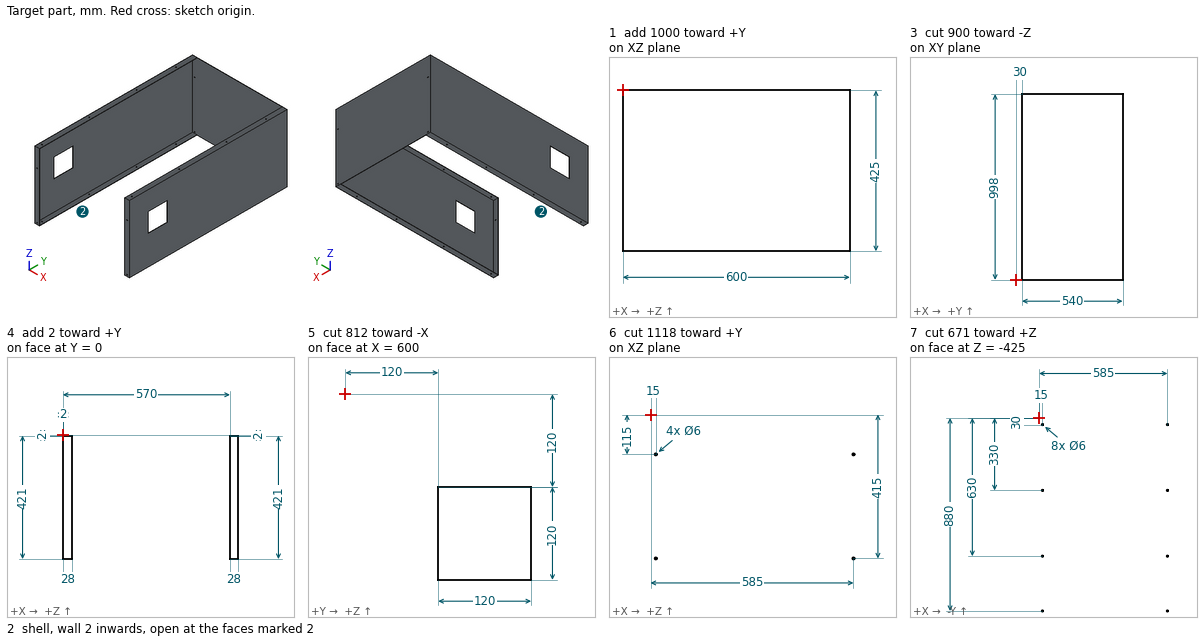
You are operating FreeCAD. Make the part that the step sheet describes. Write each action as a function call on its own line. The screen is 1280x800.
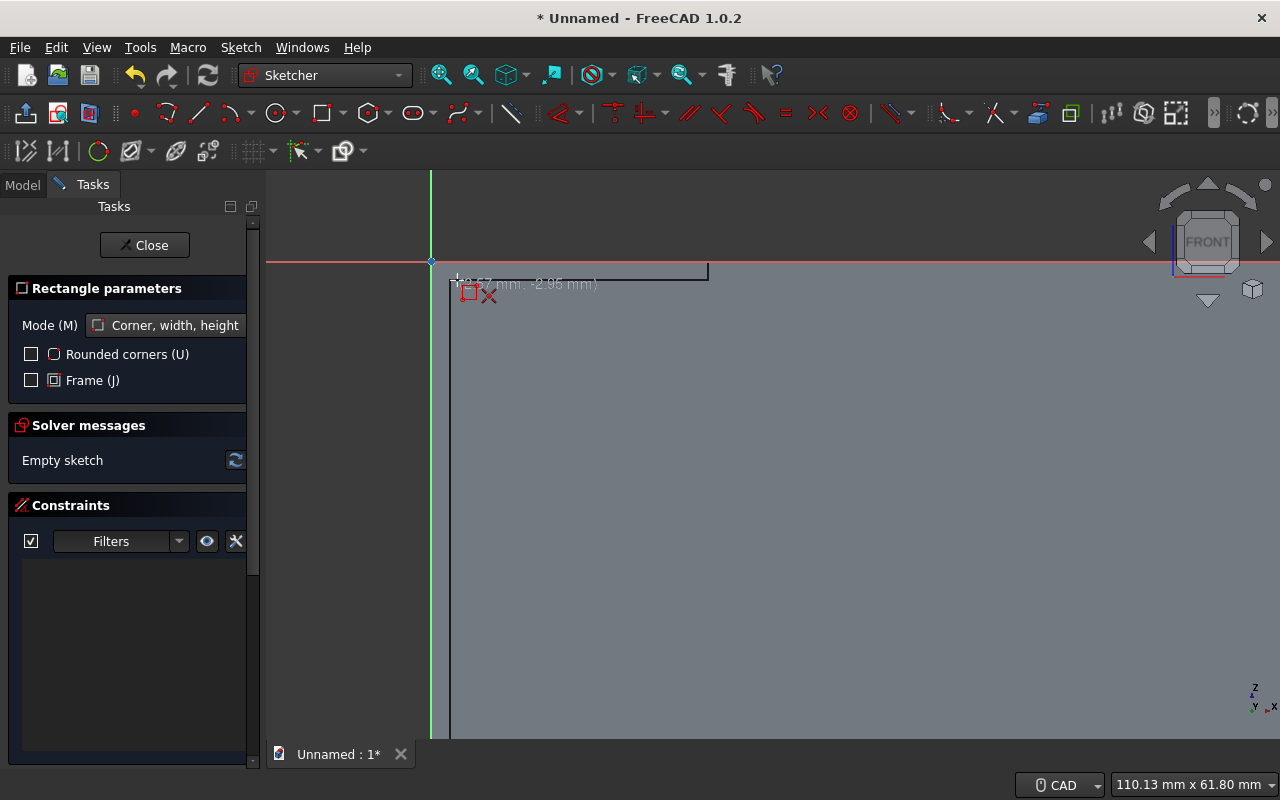
click(450, 280)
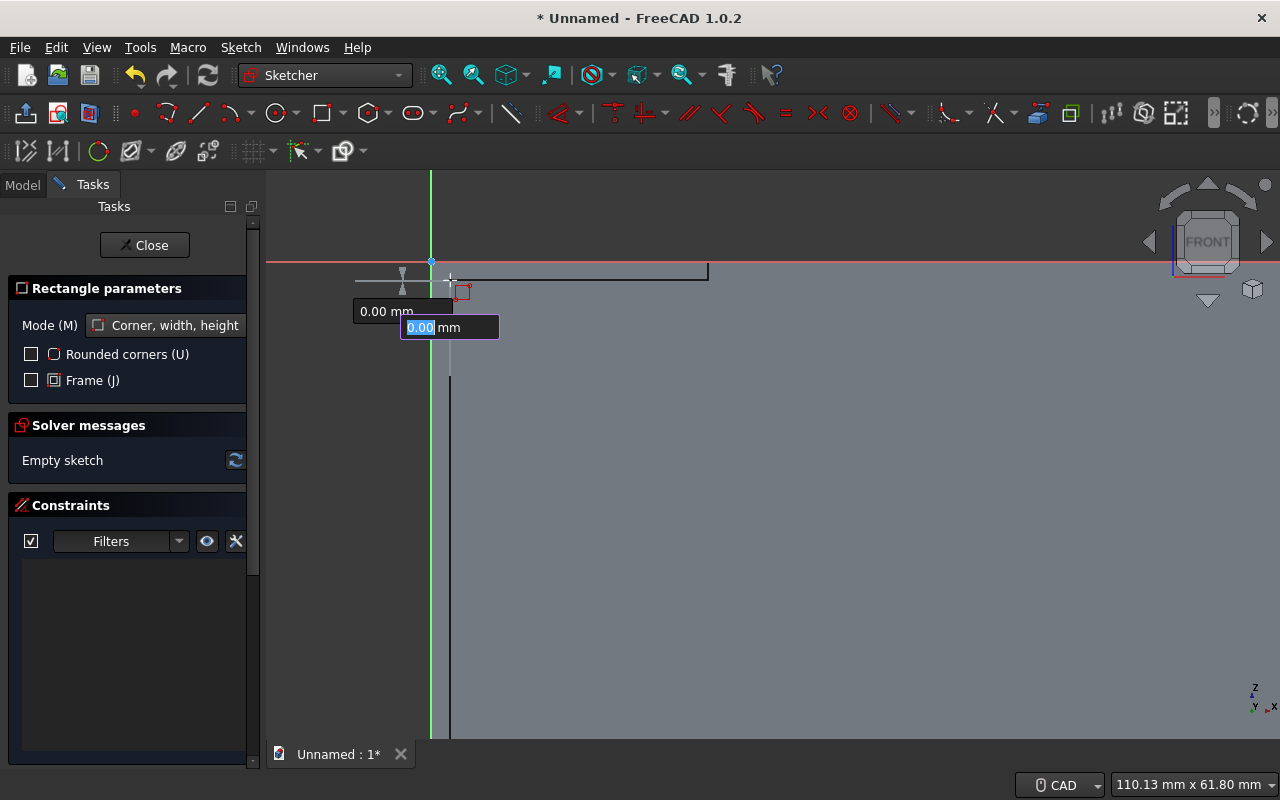
scroll(457, 279, down, 12)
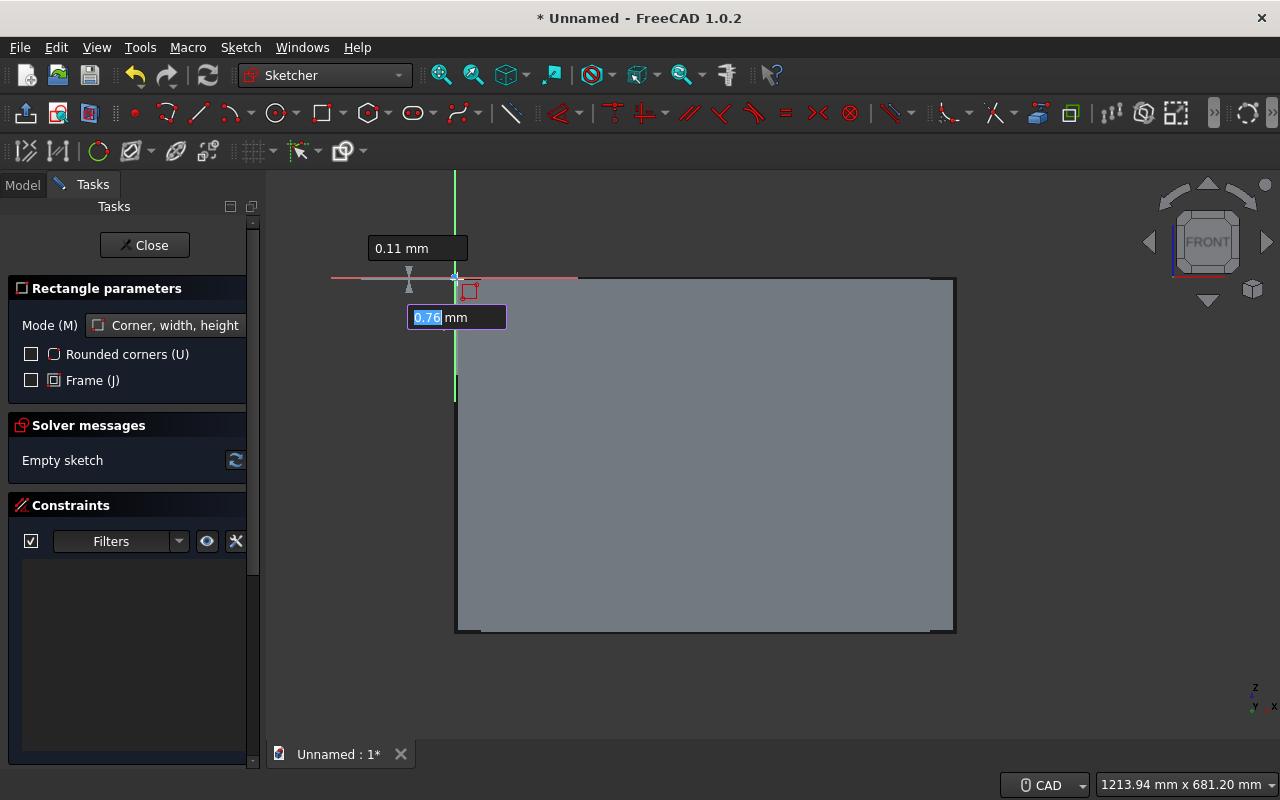
click(480, 631)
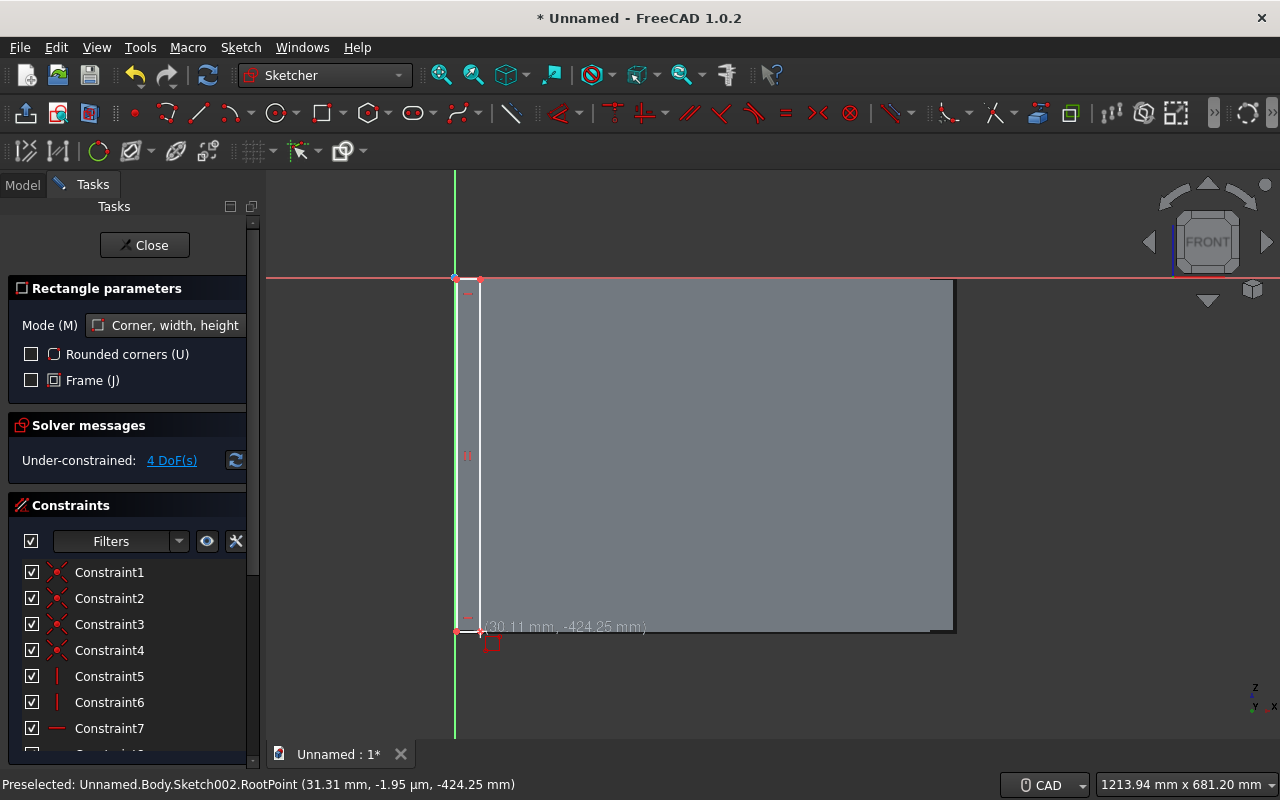
scroll(931, 279, up, 12)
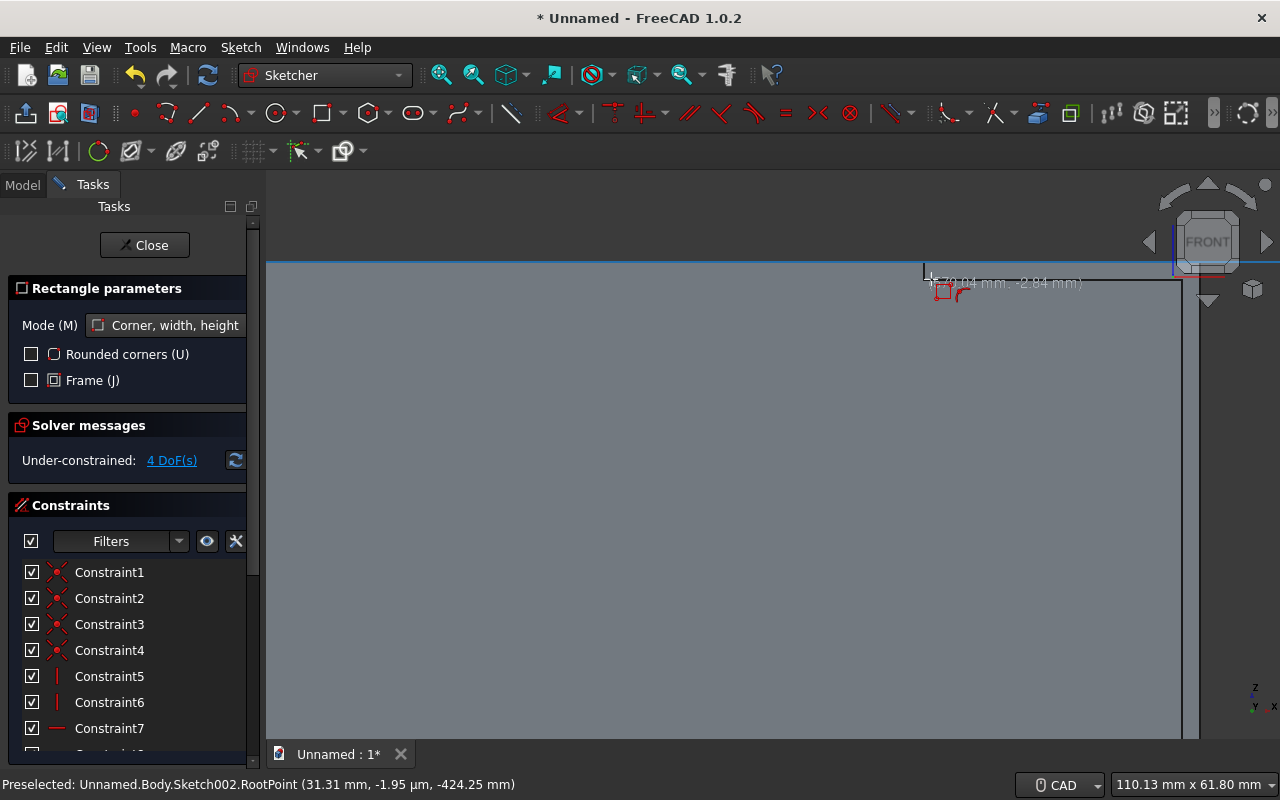
click(924, 280)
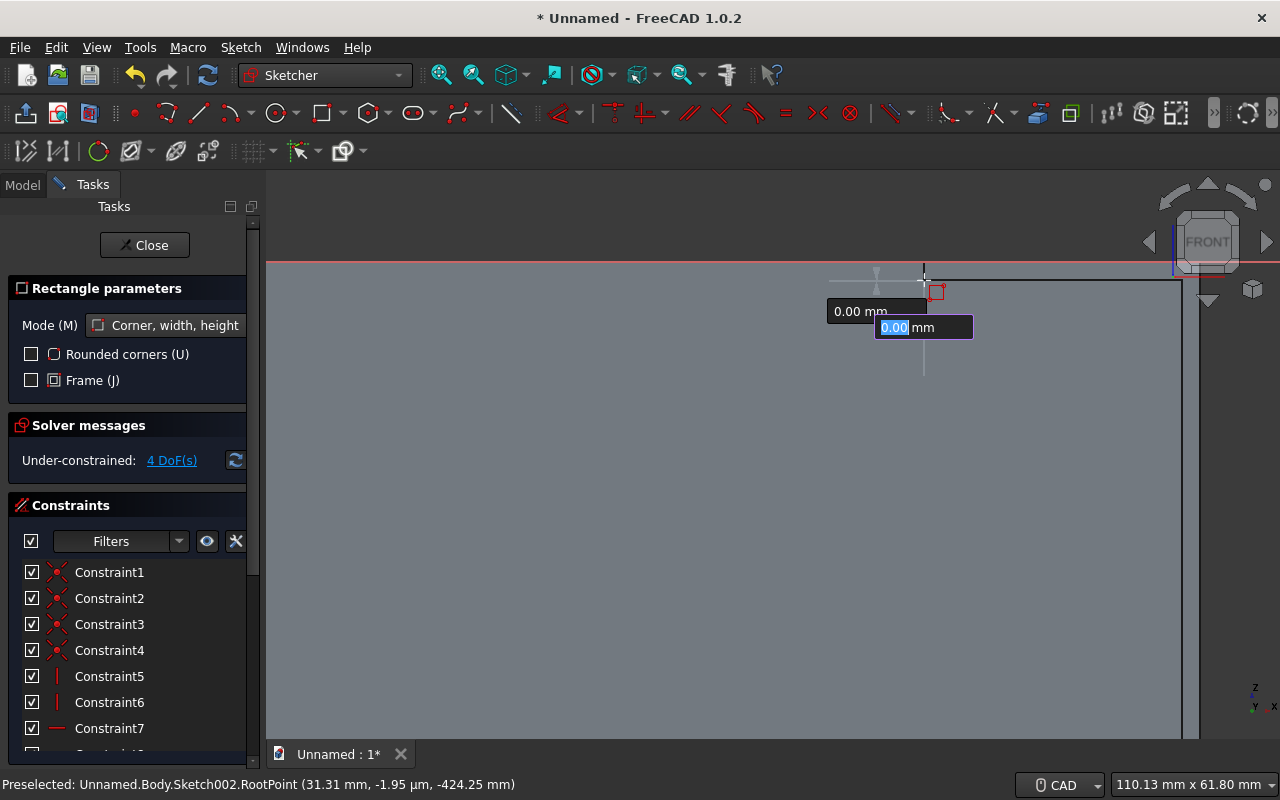
scroll(932, 279, down, 12)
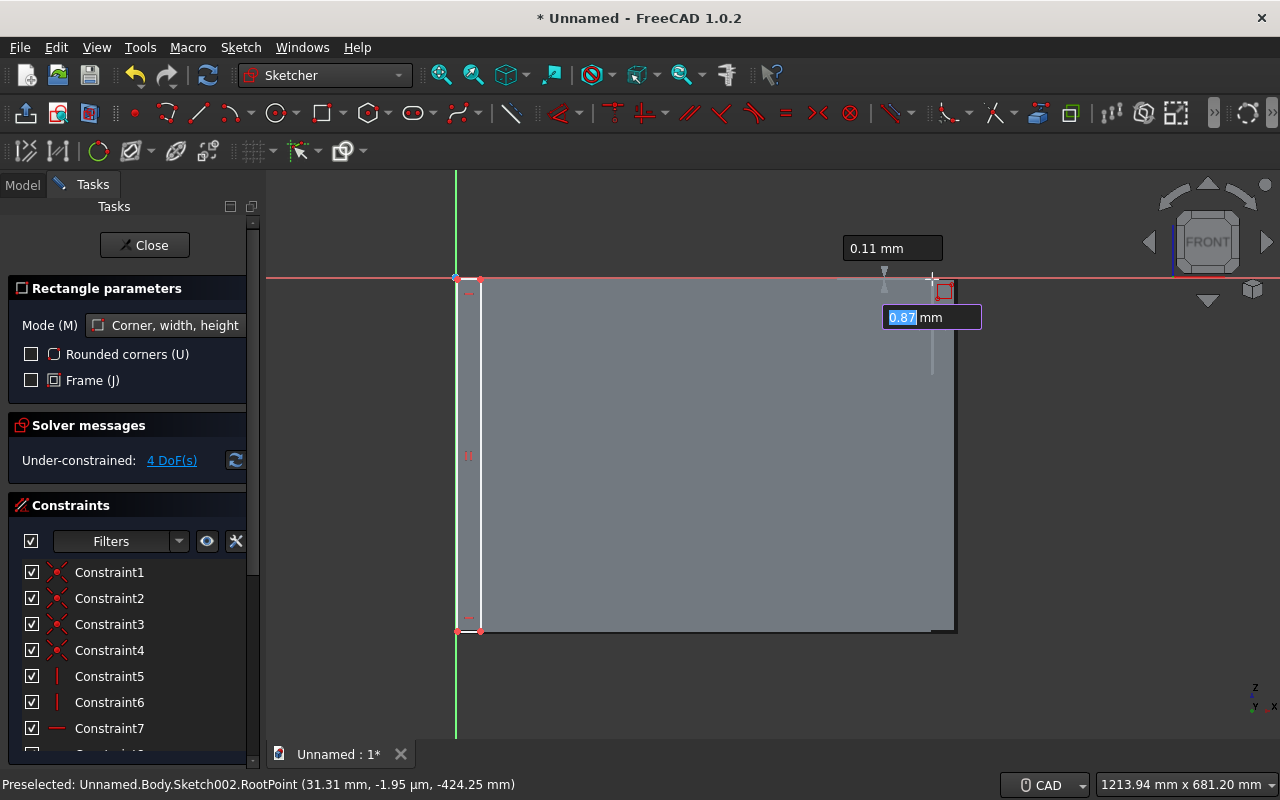
click(955, 631)
key(Escape)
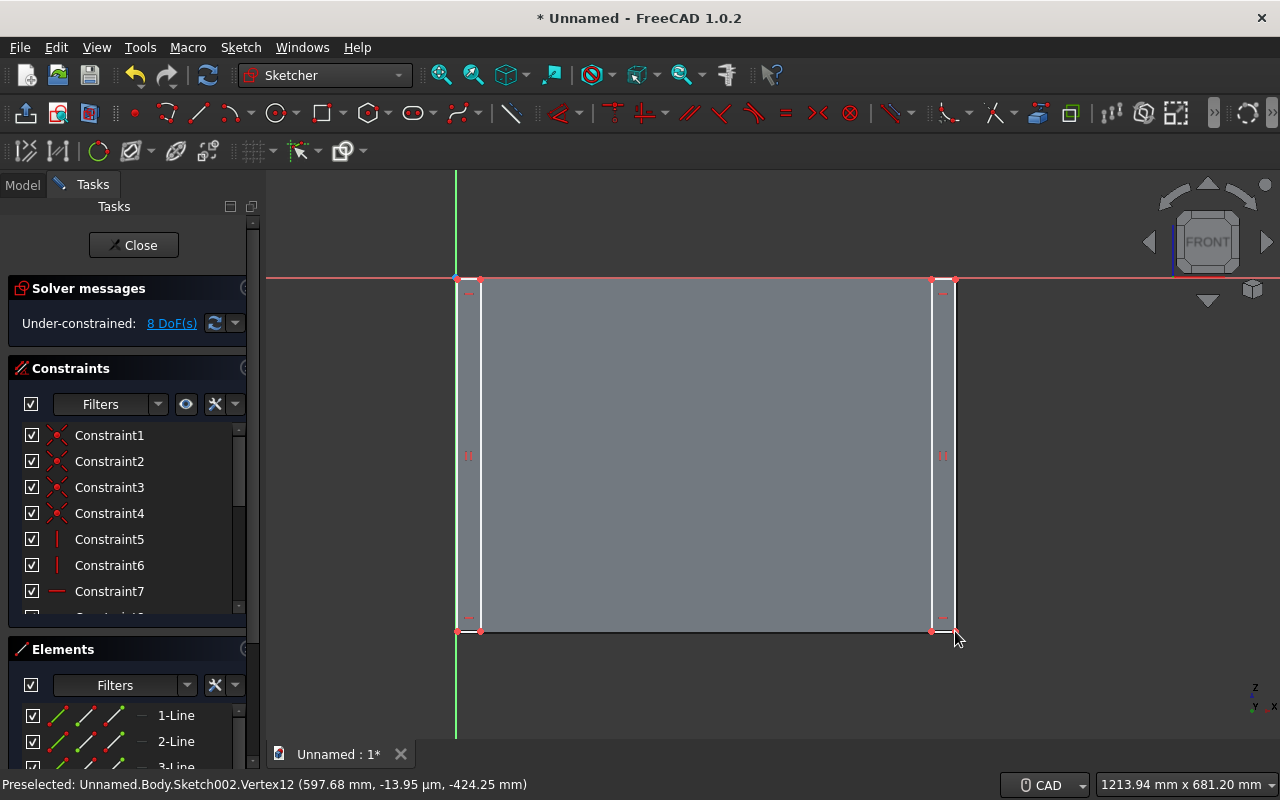
scroll(467, 632, up, 3)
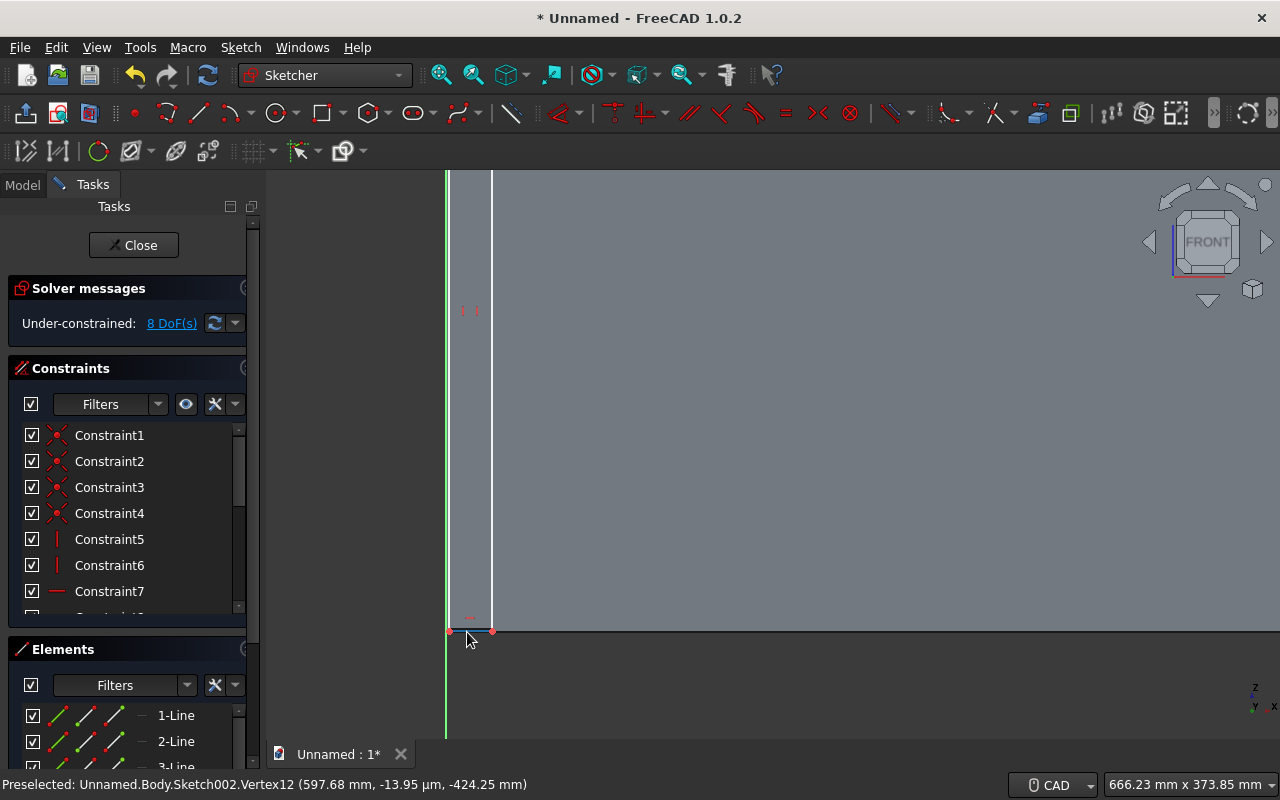
click(467, 631)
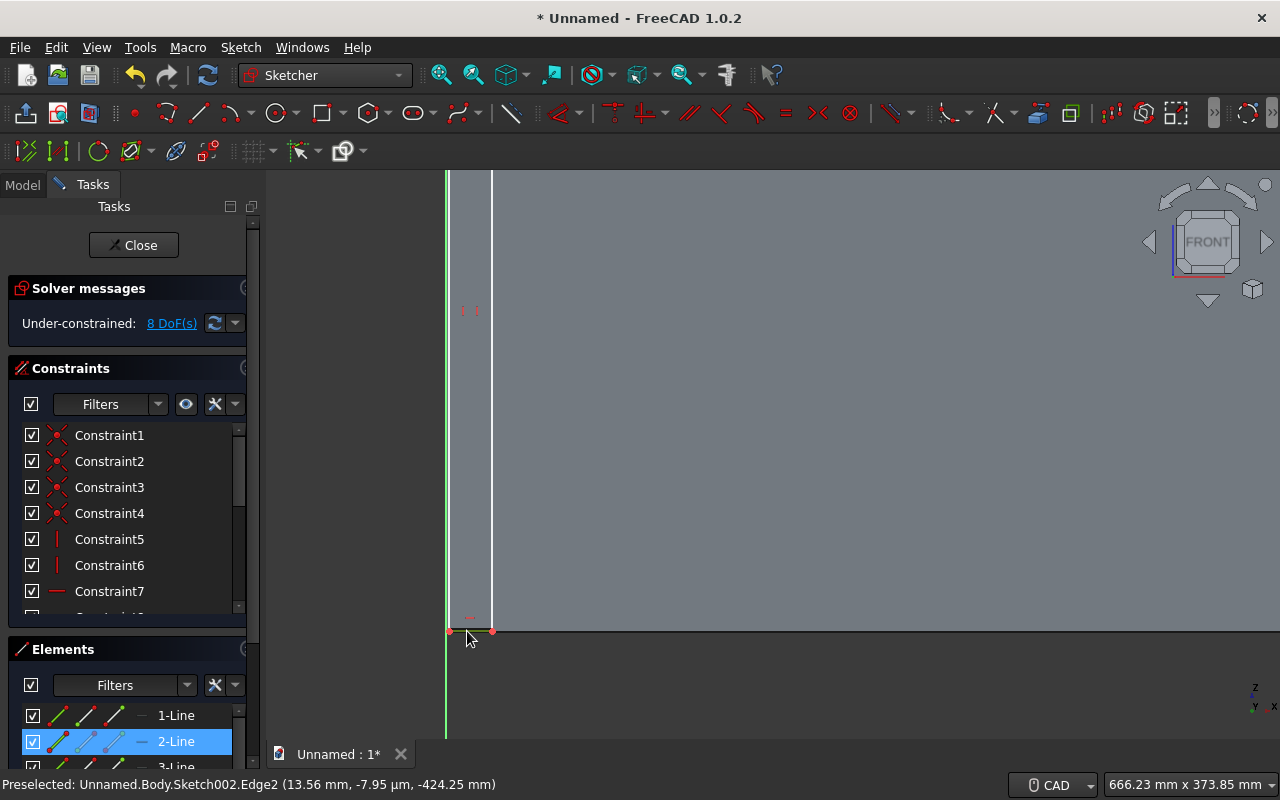
click(582, 114)